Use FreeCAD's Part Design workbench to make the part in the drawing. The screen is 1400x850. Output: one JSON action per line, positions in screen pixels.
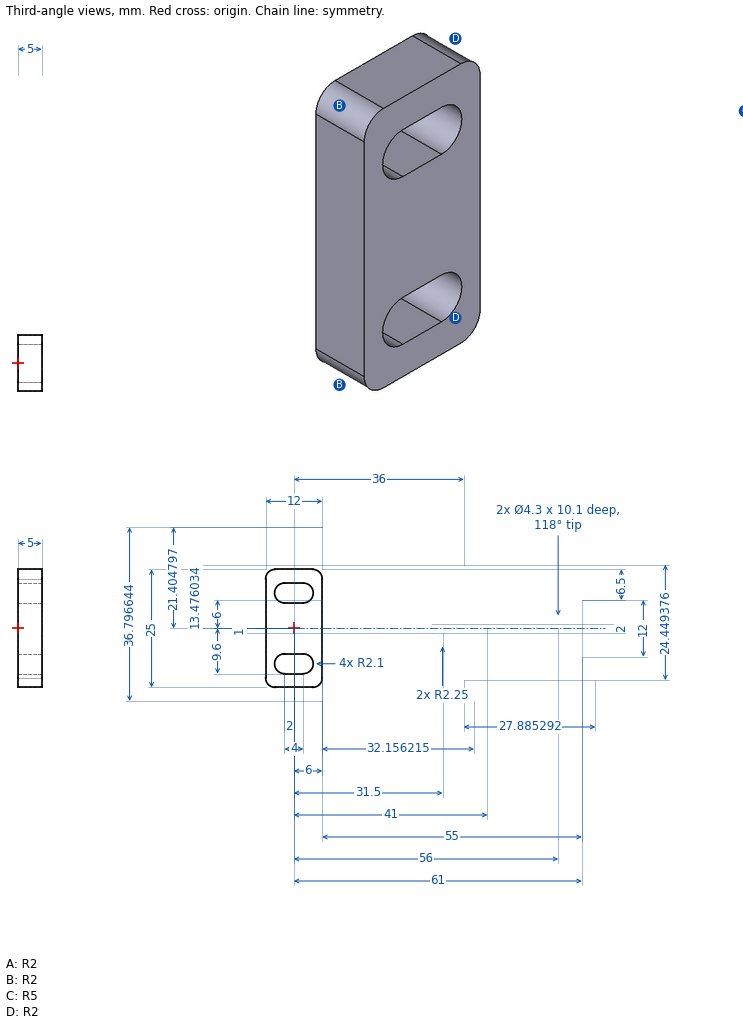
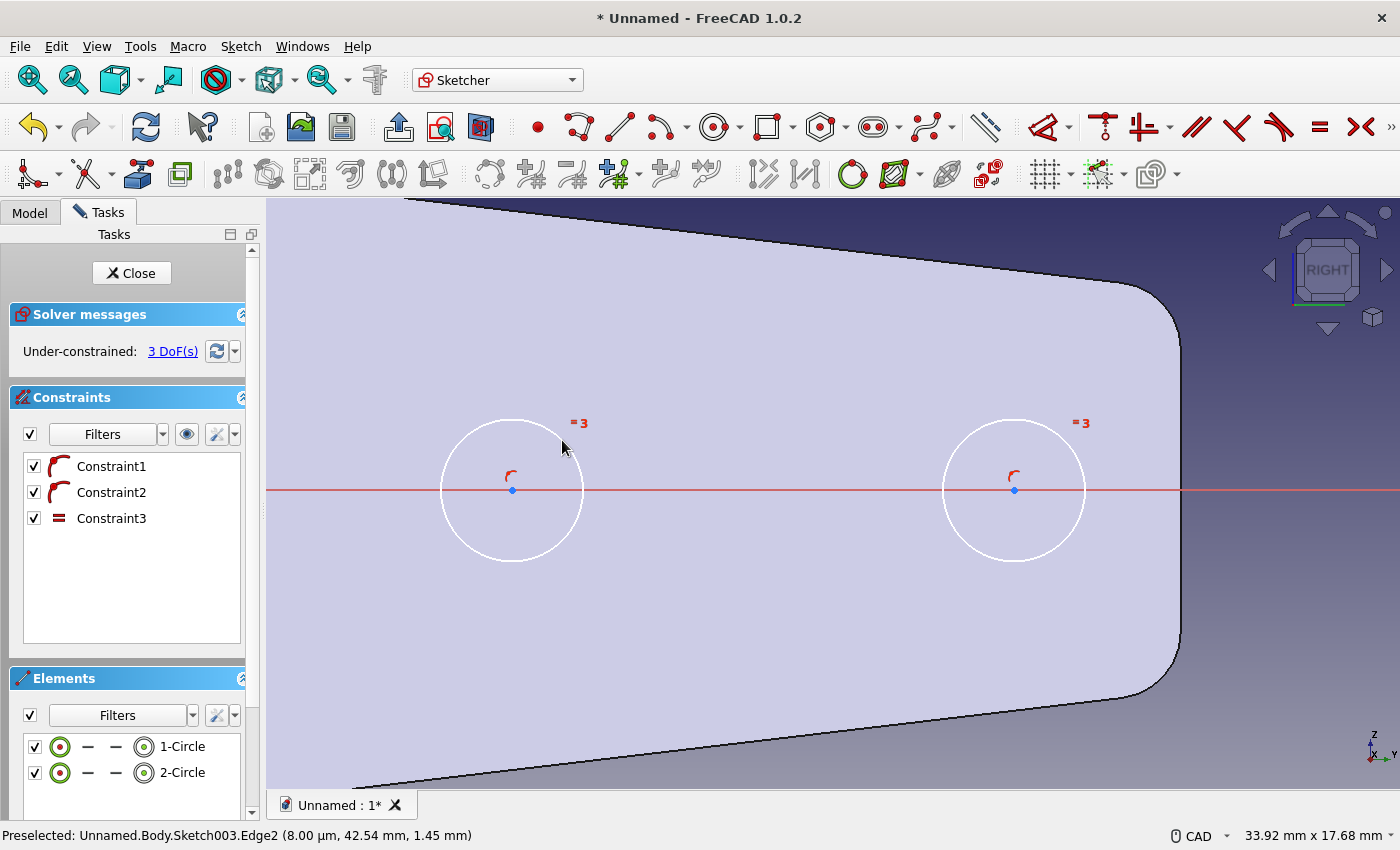
{"action": "left_click", "coordinate": [1042, 128]}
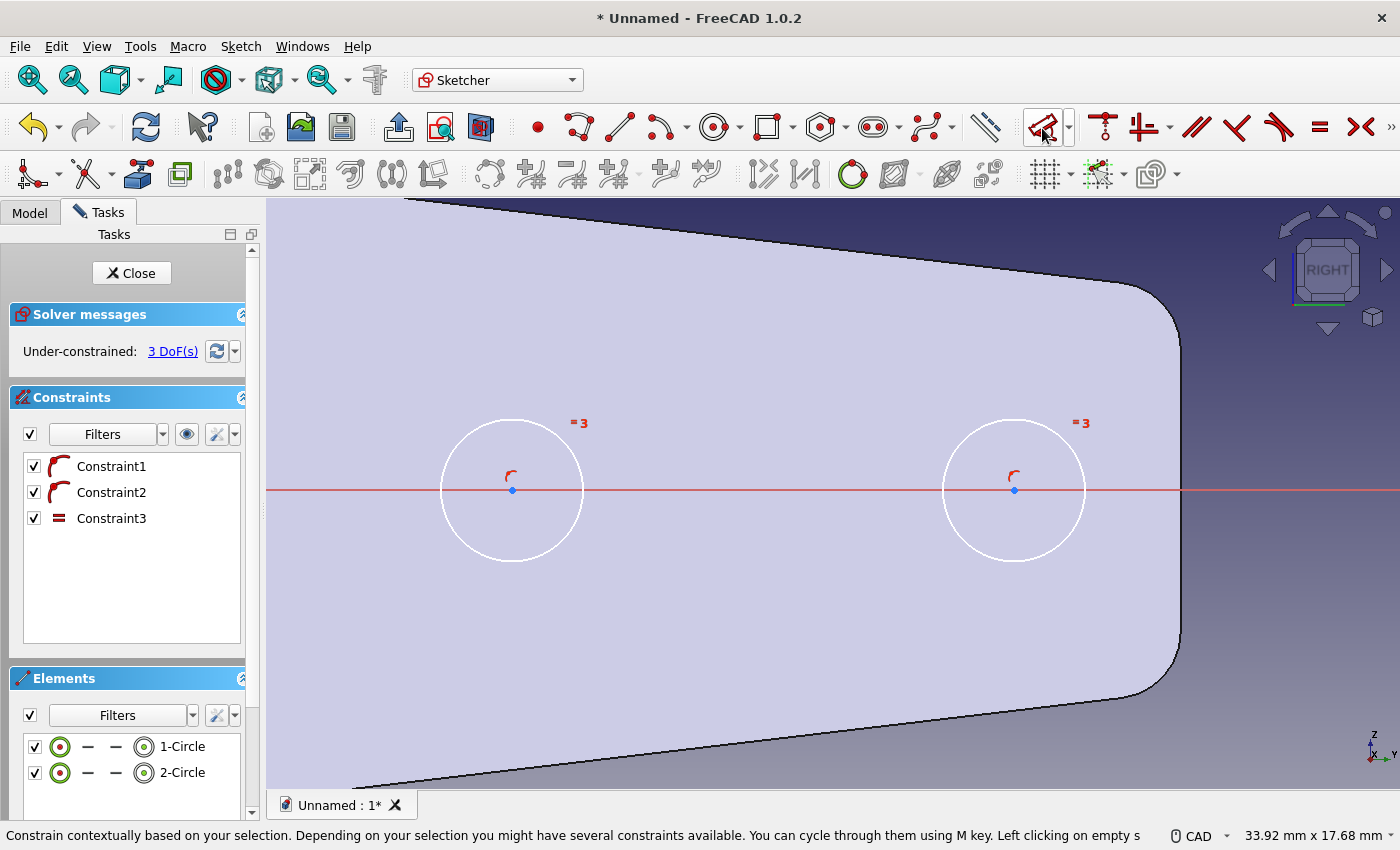
{"action": "left_click", "coordinate": [1064, 440]}
{"action": "left_click", "coordinate": [1087, 417]}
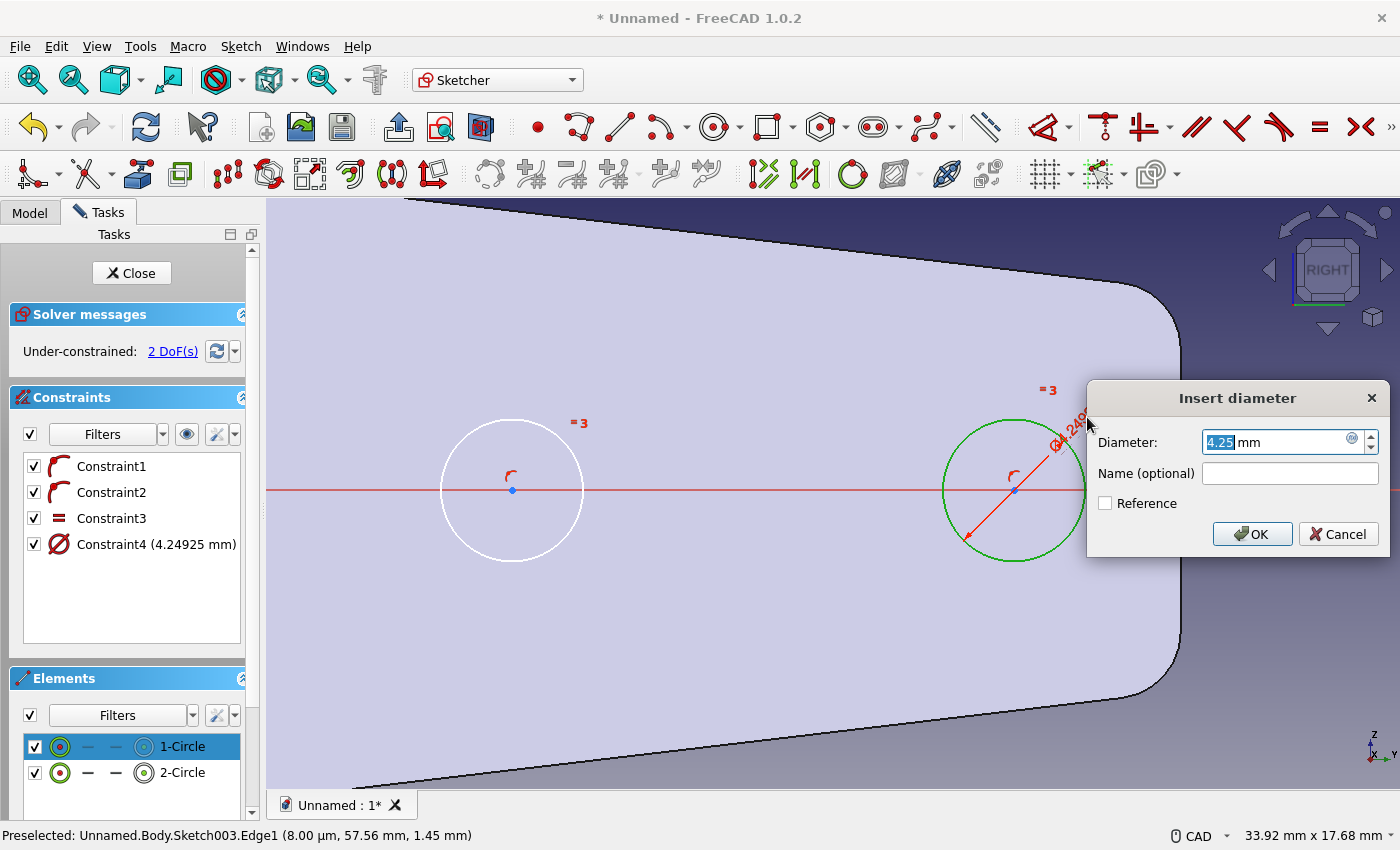
{"action": "type", "text": "4.3"}
{"action": "key", "text": "Return"}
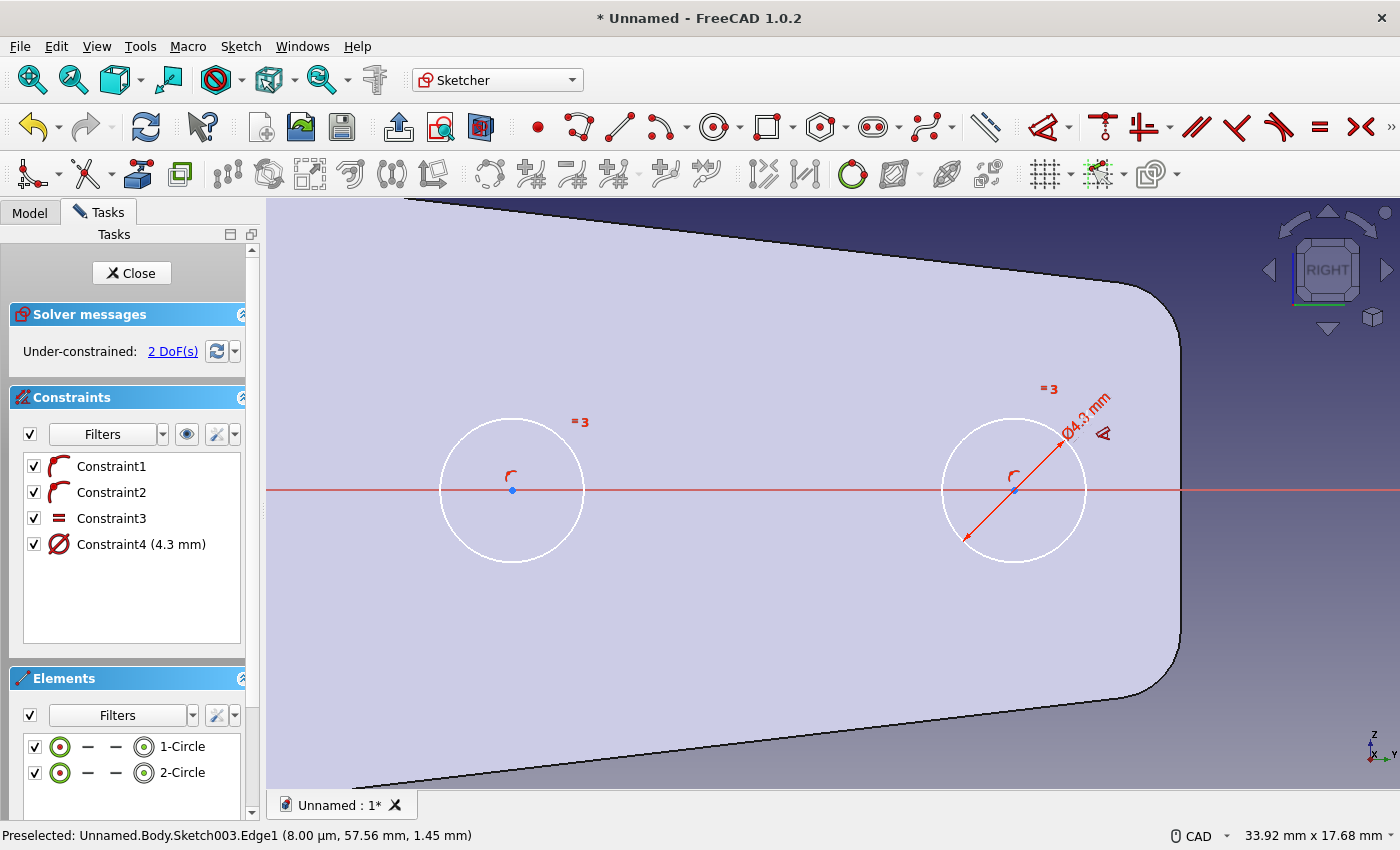
{"action": "left_click", "coordinate": [1014, 490]}
{"action": "left_click", "coordinate": [654, 524]}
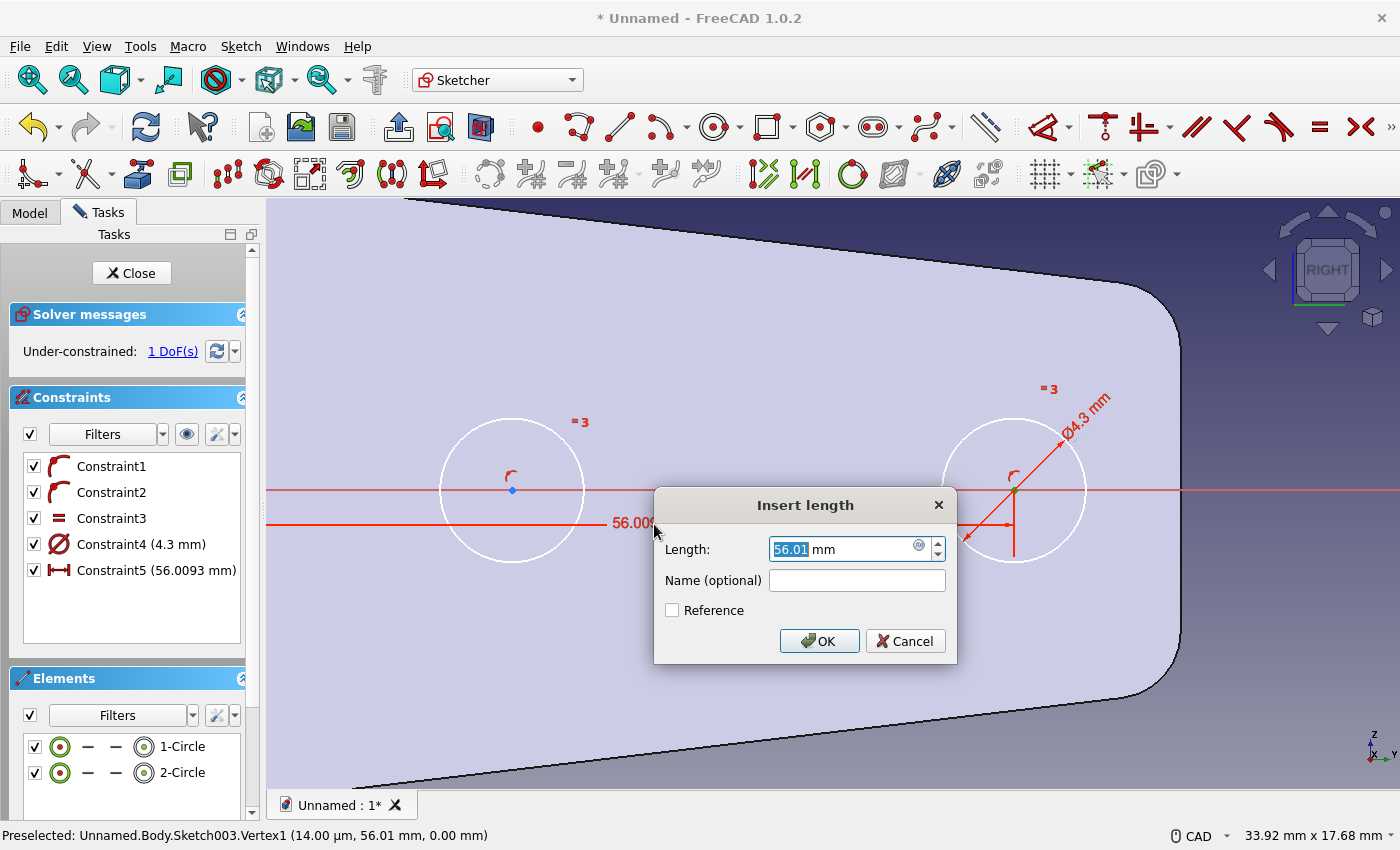
{"action": "type", "text": "56"}
{"action": "key", "text": "Return"}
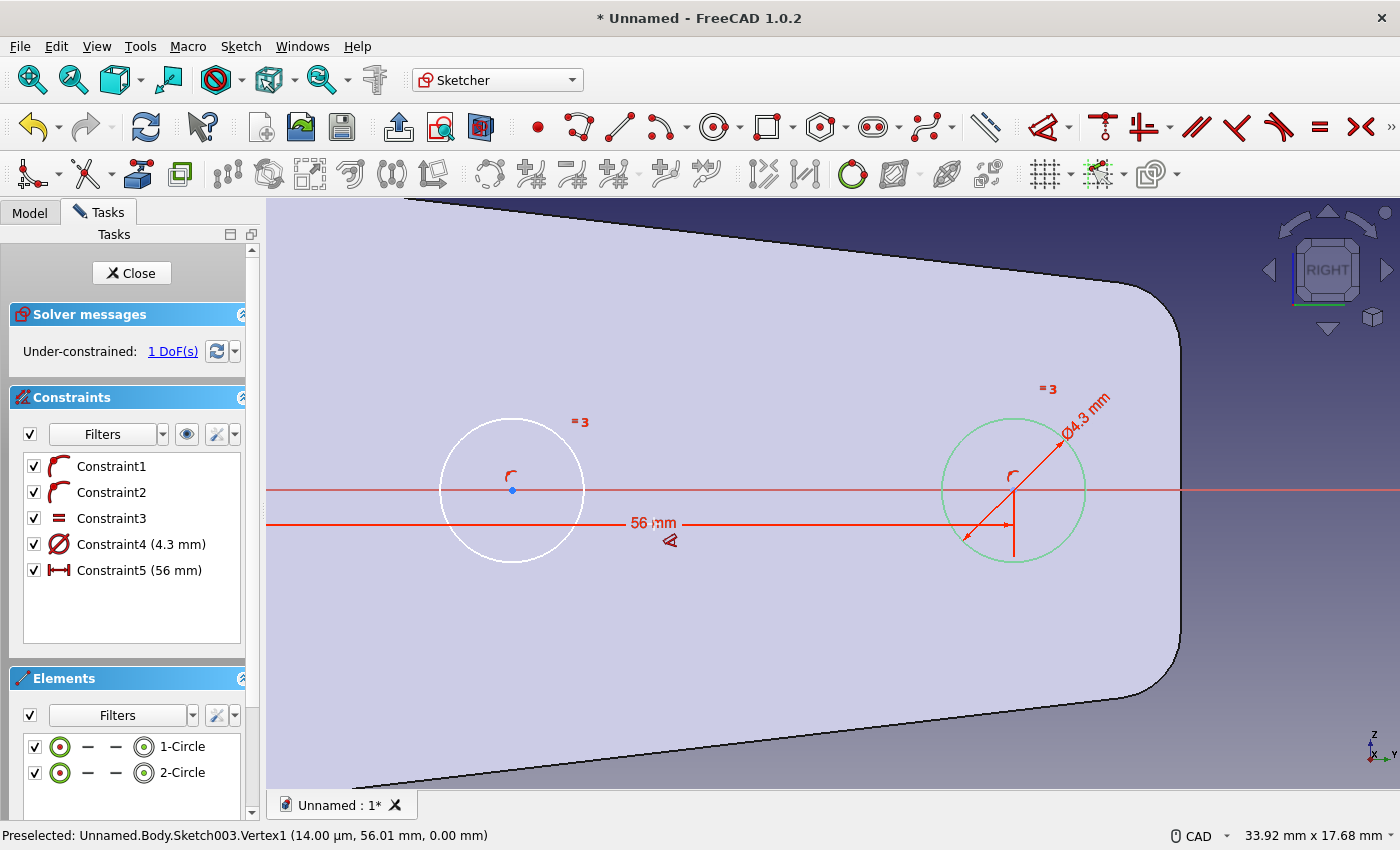
{"action": "left_click", "coordinate": [512, 490]}
{"action": "left_click", "coordinate": [403, 524]}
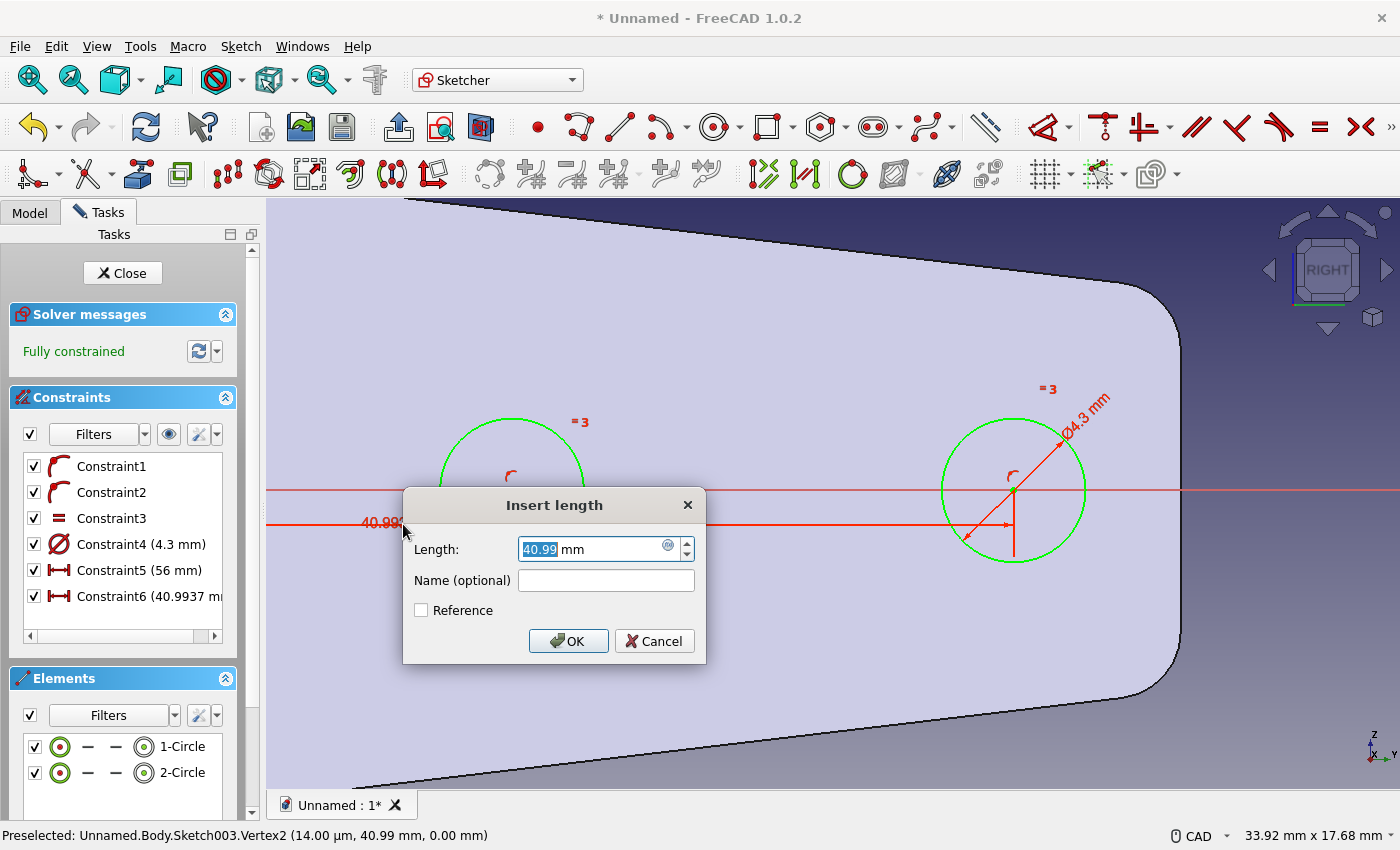
{"action": "type", "text": "41"}
{"action": "key", "text": "Return"}
{"action": "key", "text": "Escape"}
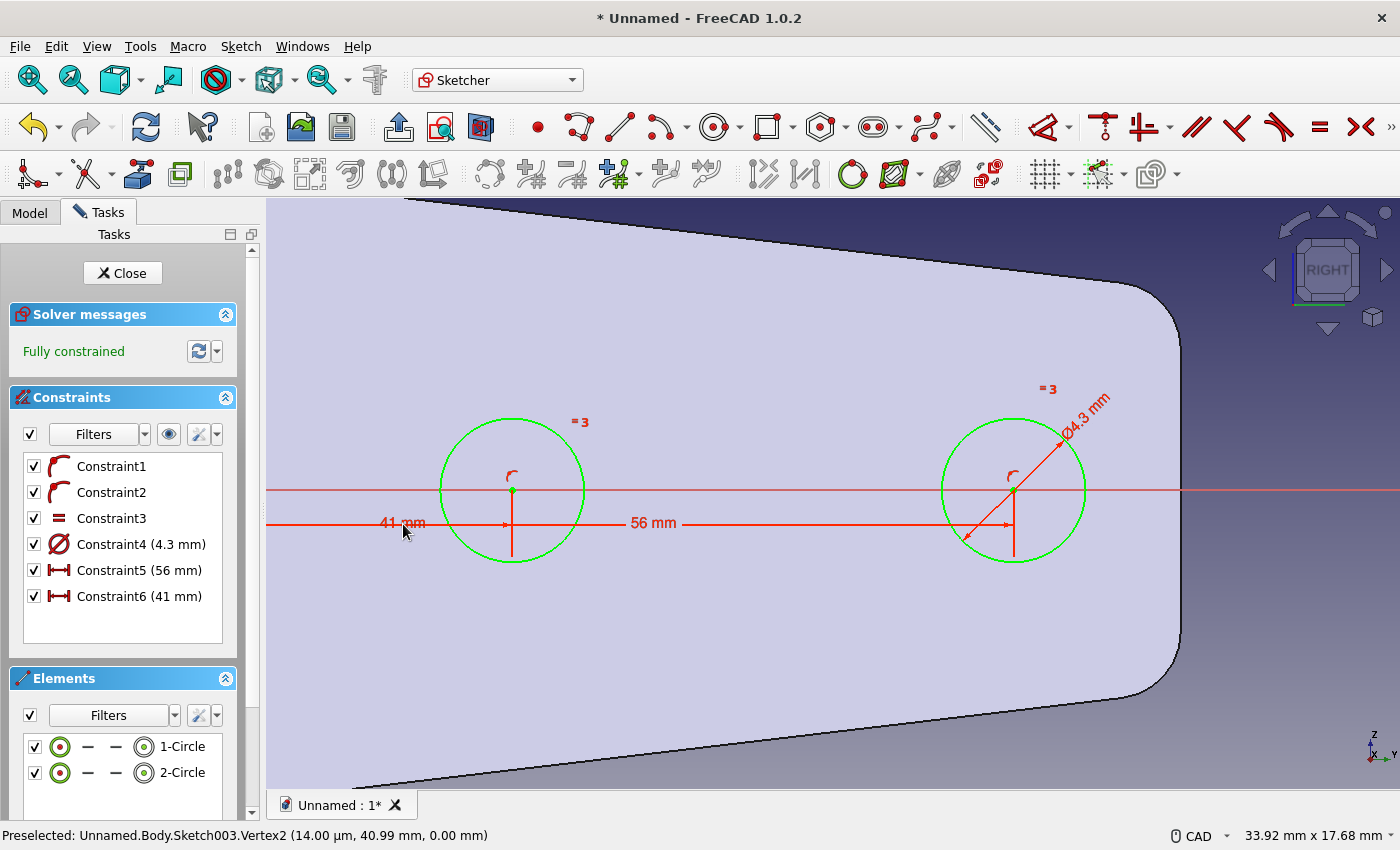
{"action": "left_click", "coordinate": [123, 273]}